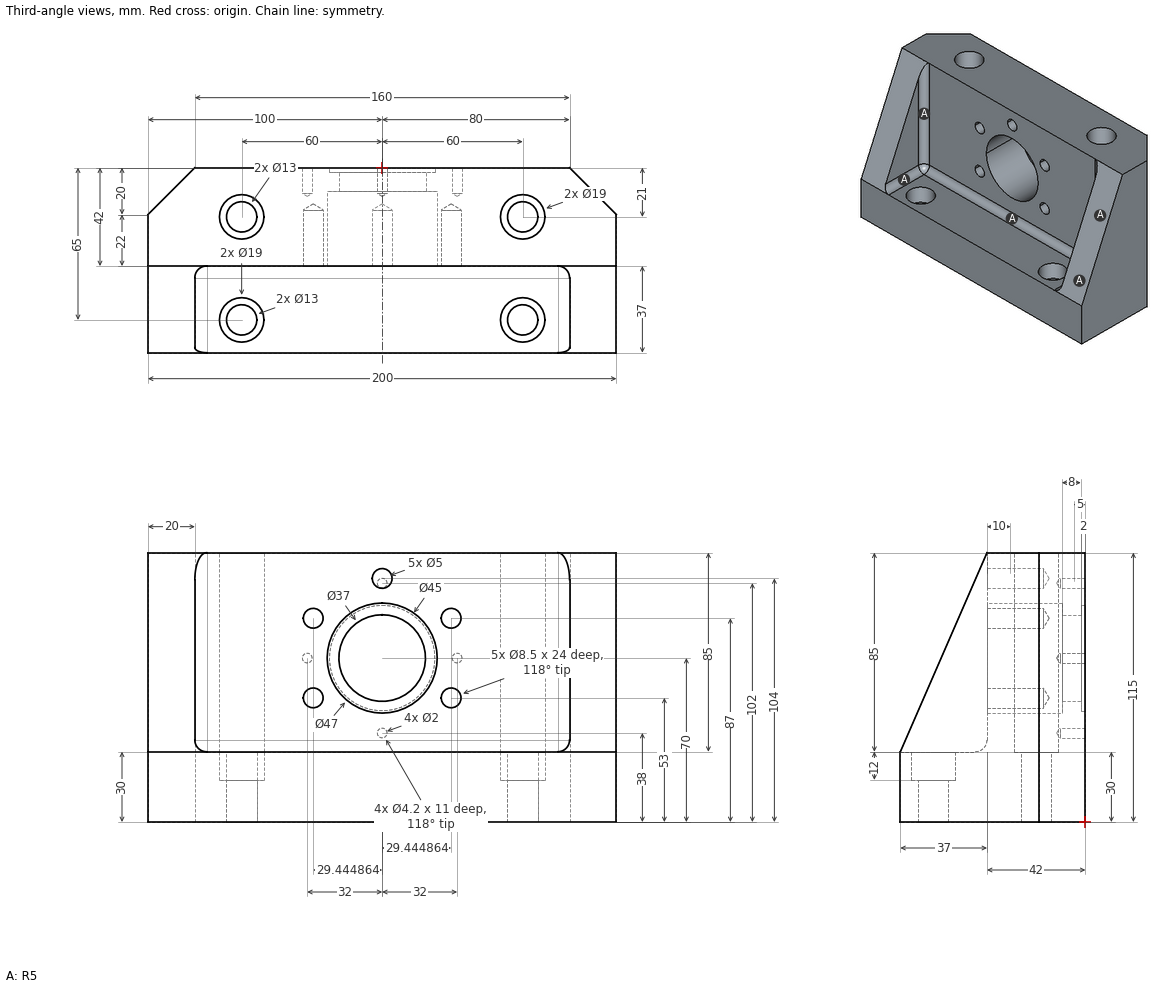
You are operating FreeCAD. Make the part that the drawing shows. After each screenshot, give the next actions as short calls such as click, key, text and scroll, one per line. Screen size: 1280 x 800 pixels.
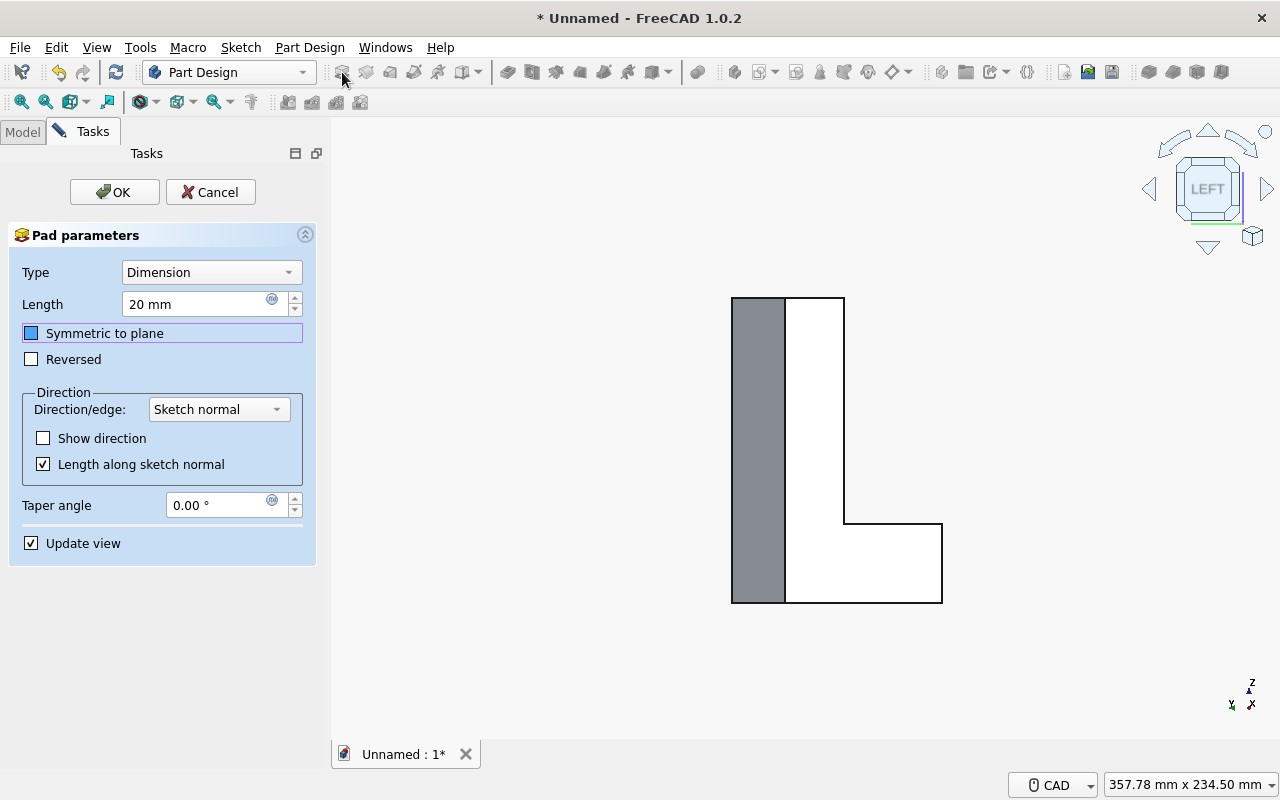
click(30, 359)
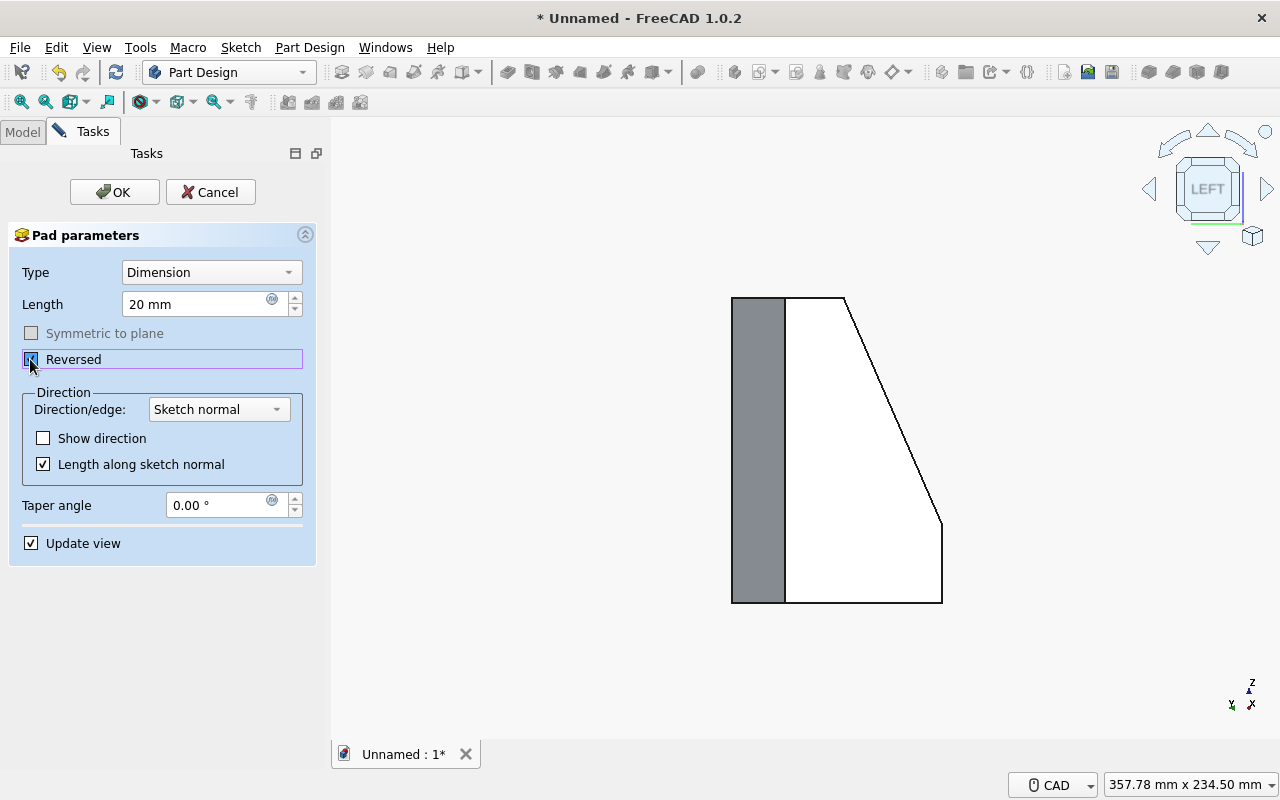
click(115, 192)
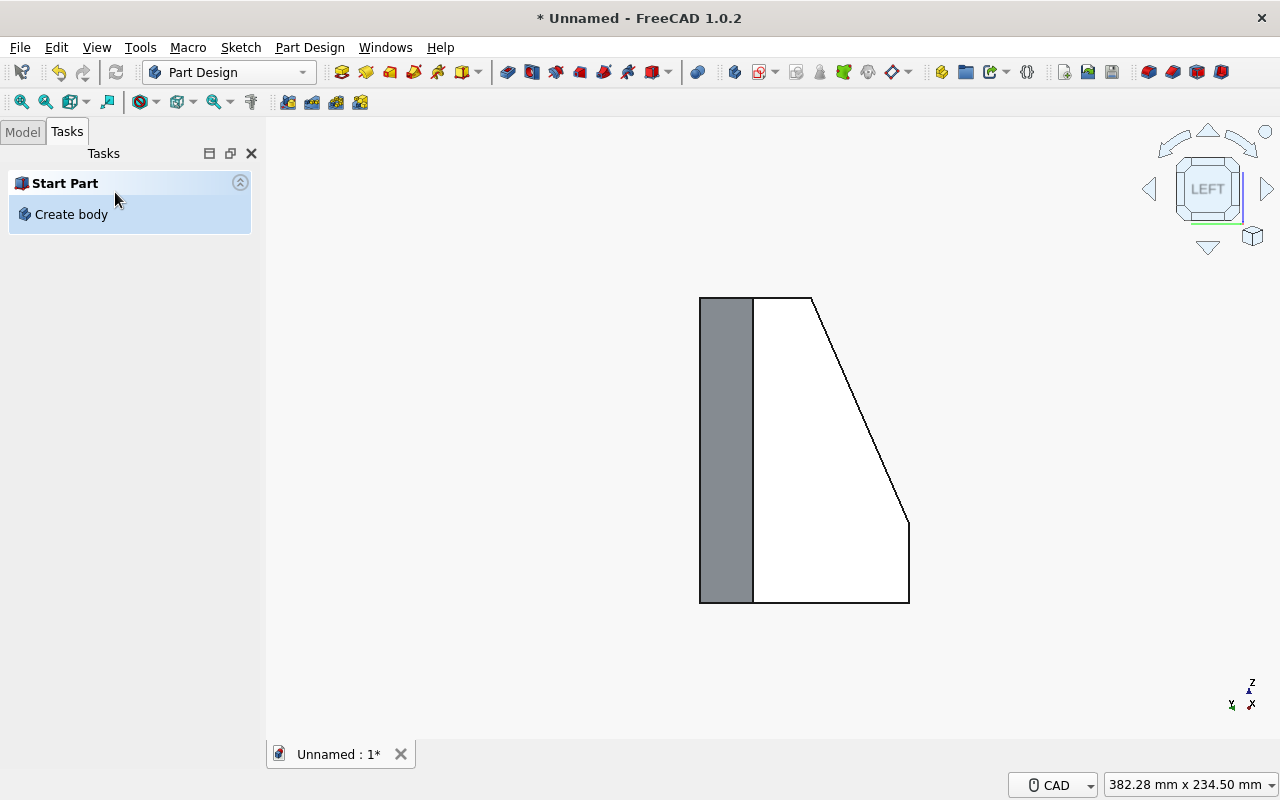
click(23, 131)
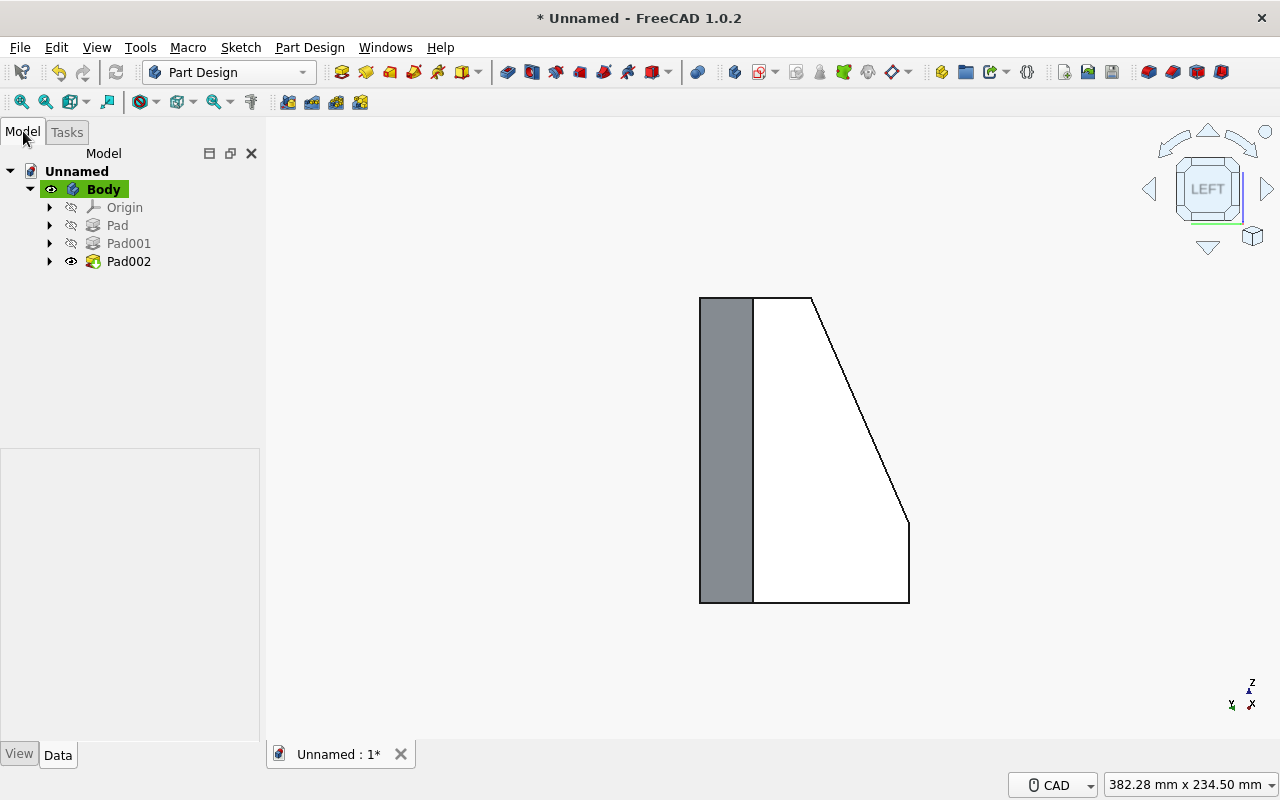
click(116, 261)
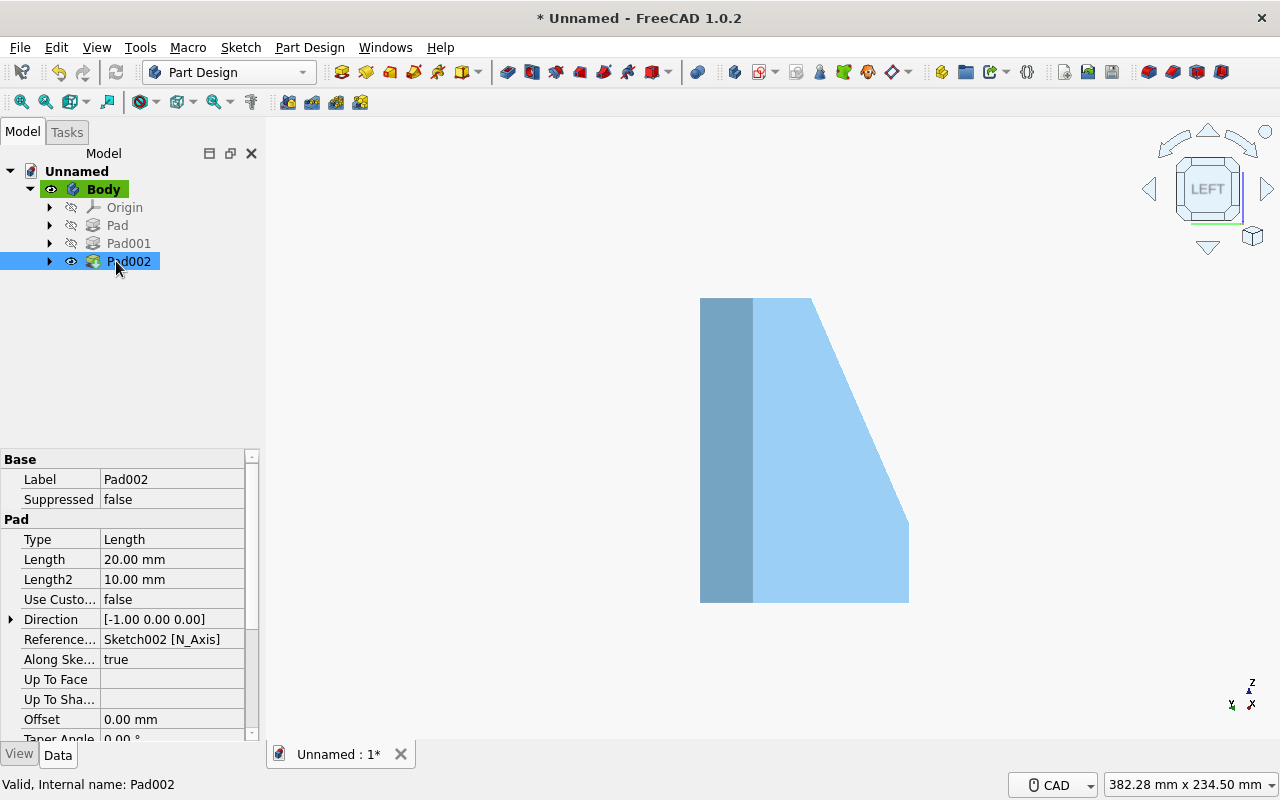
click(288, 102)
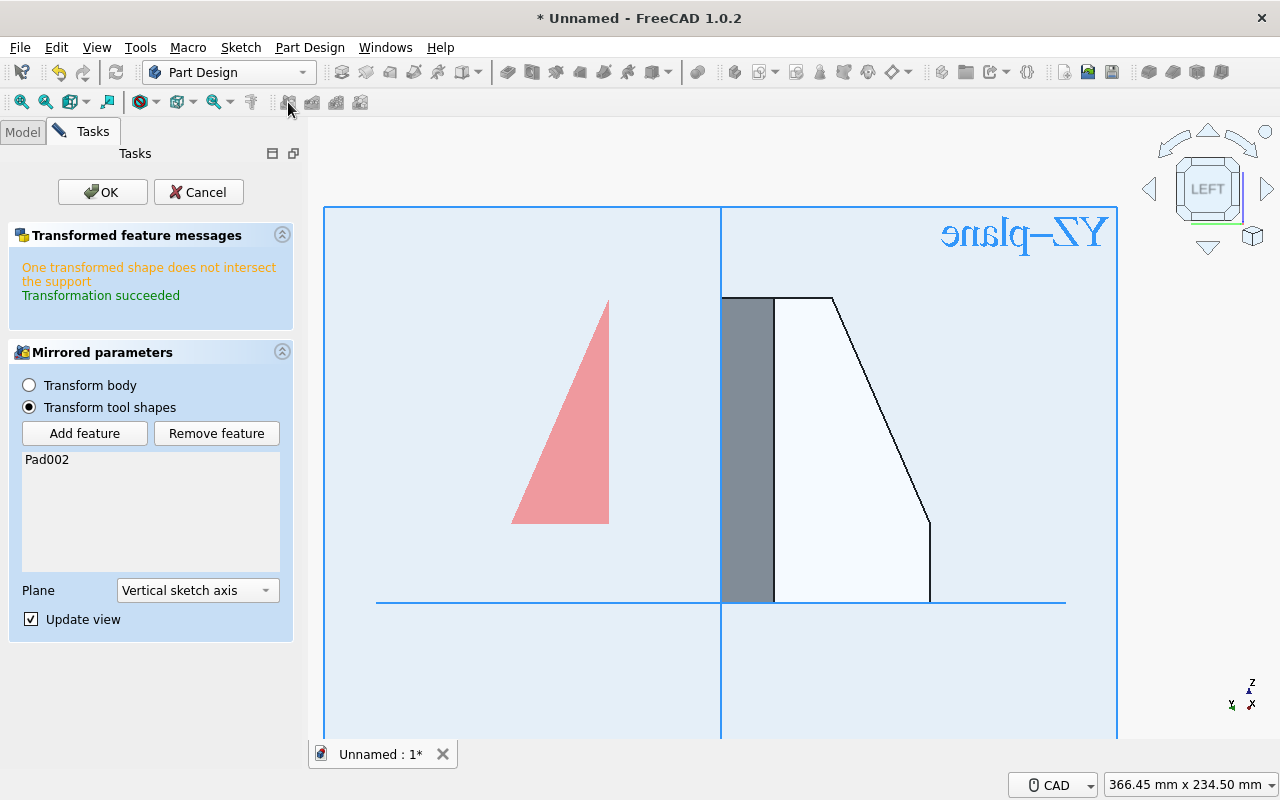
click(198, 590)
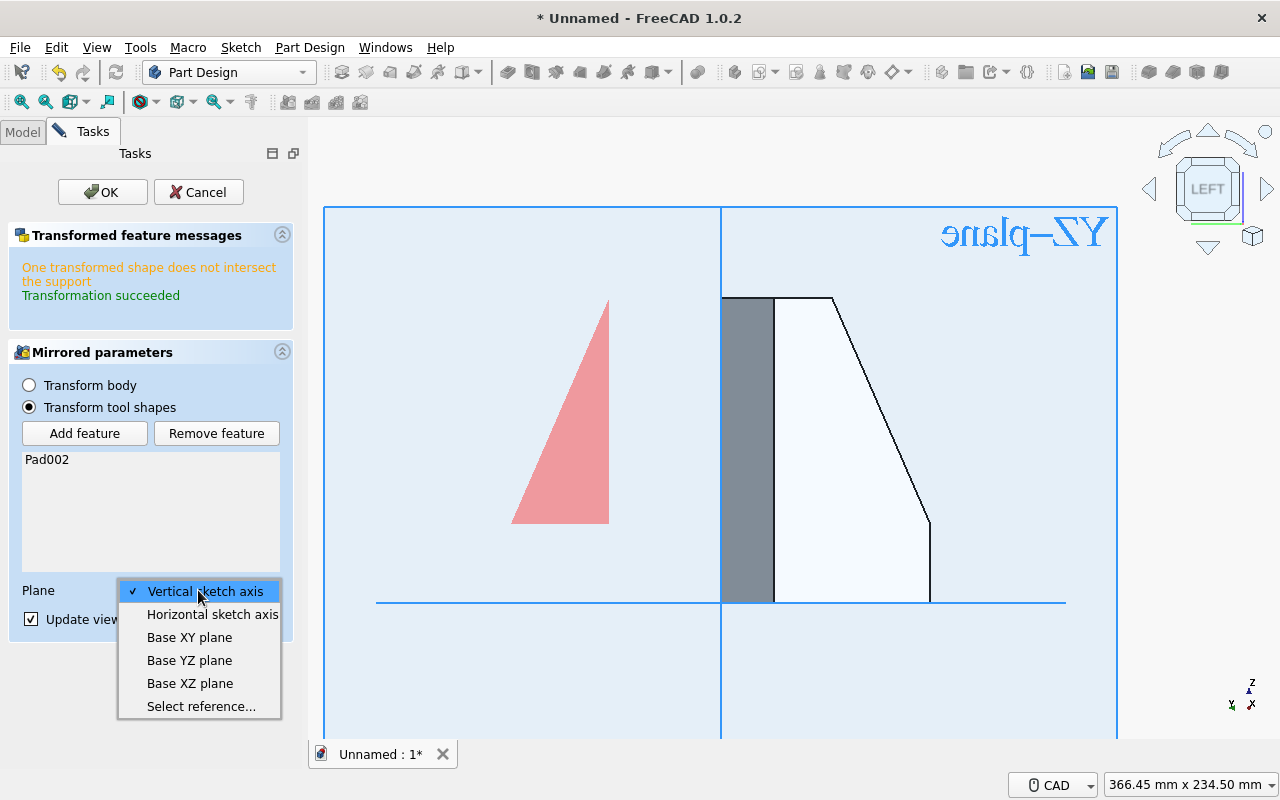
click(198, 660)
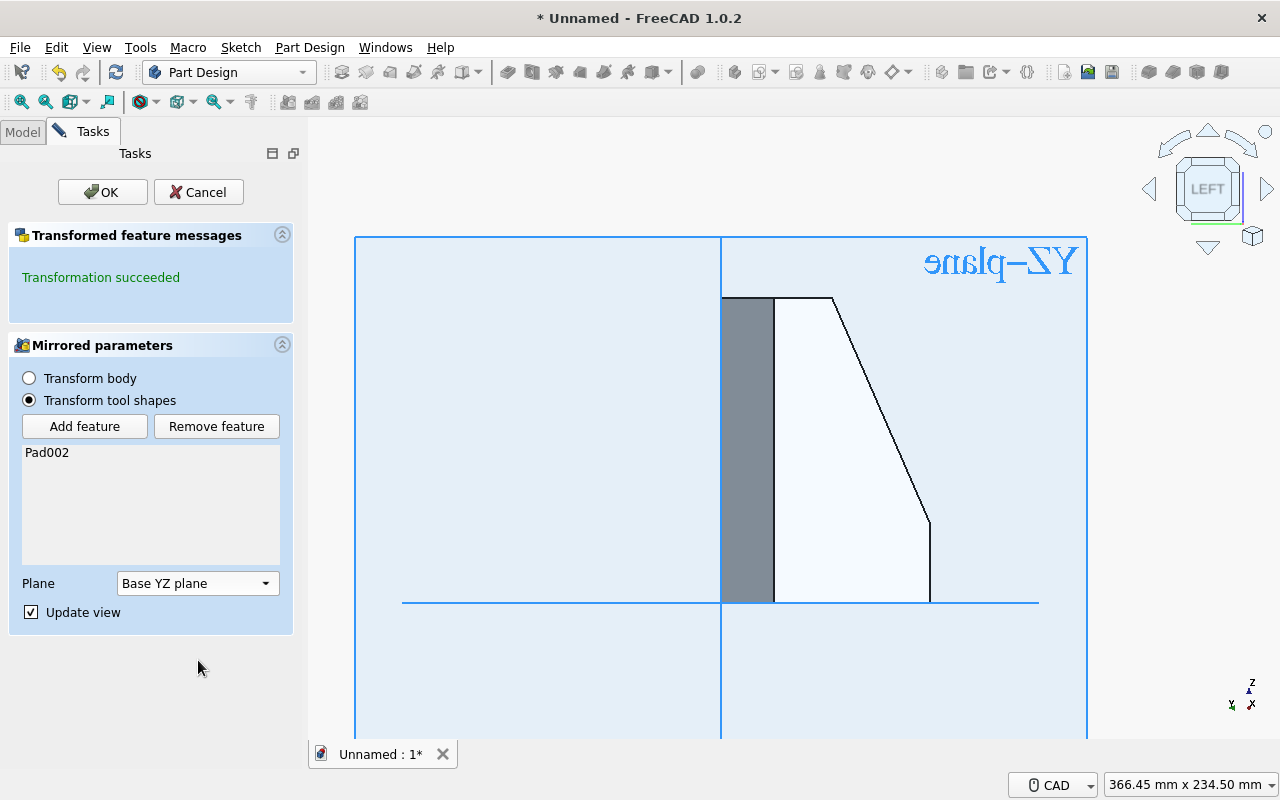
click(103, 192)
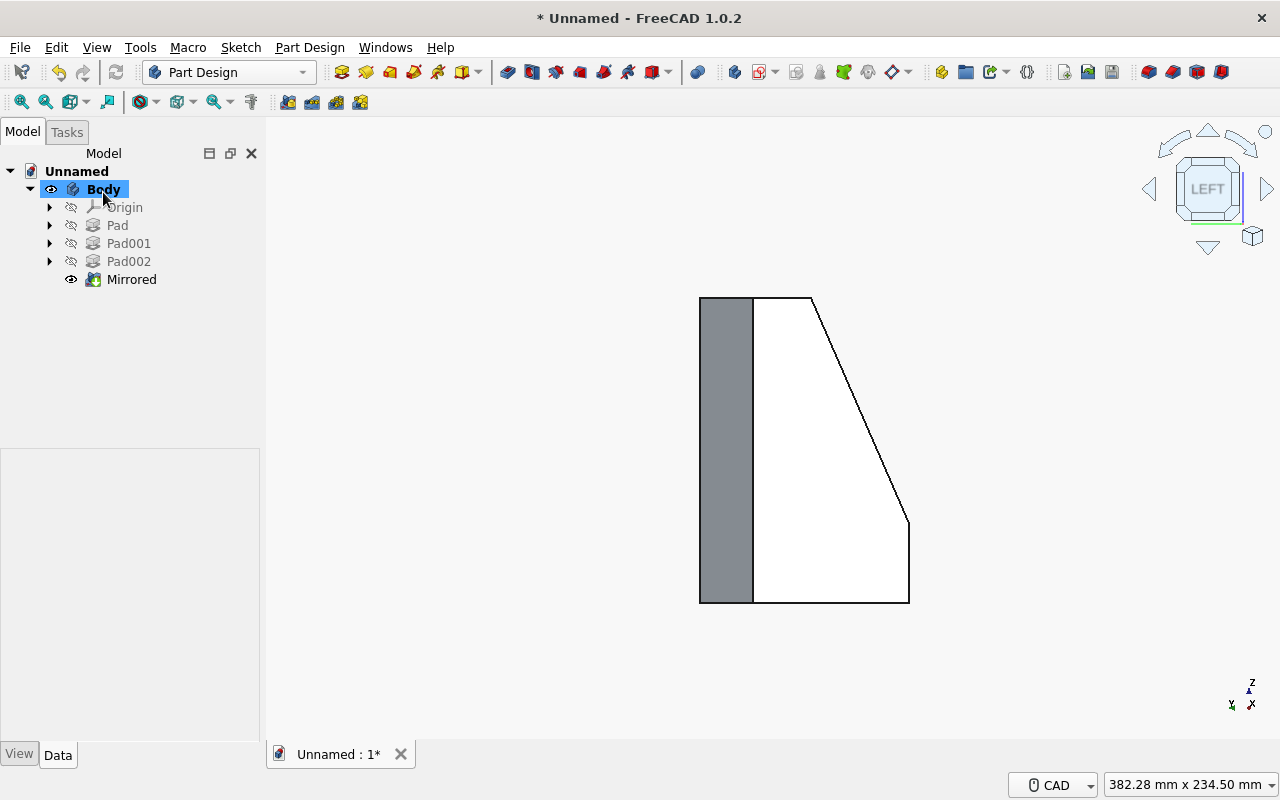
click(760, 72)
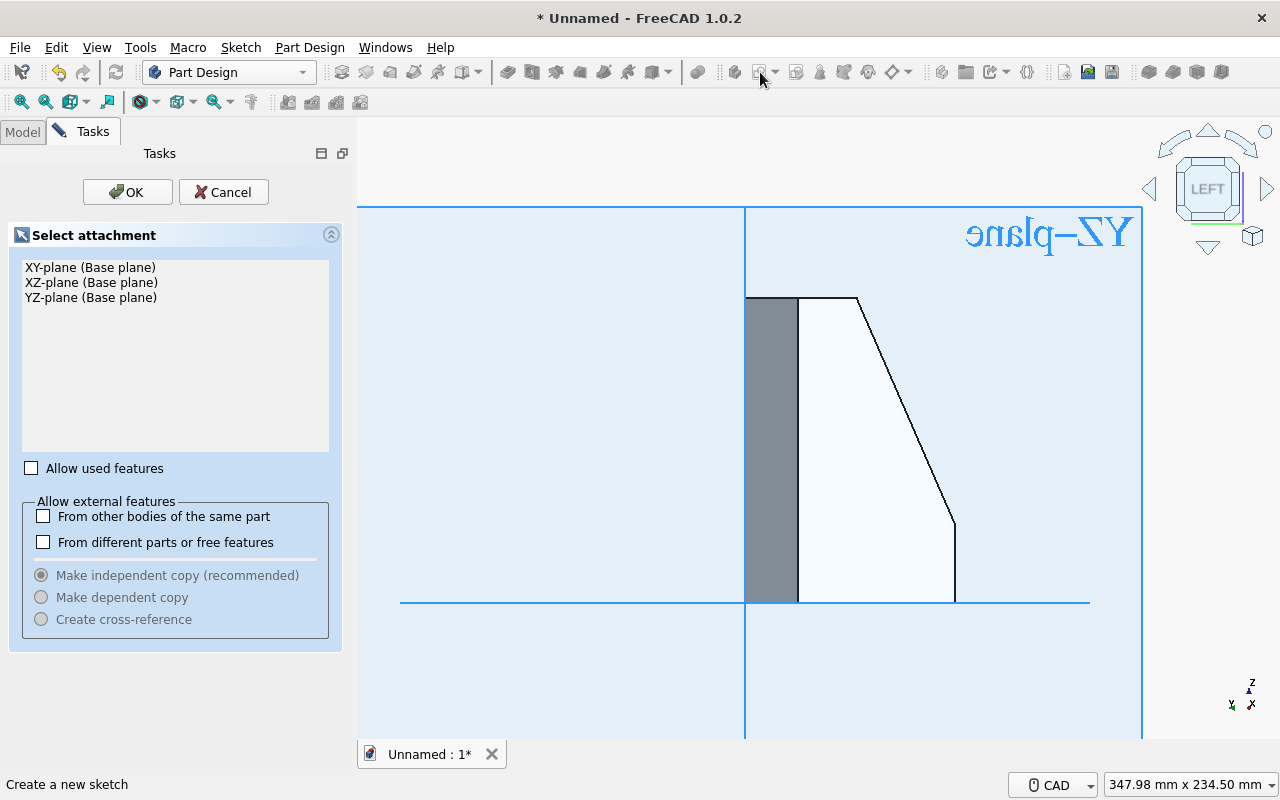
click(82, 282)